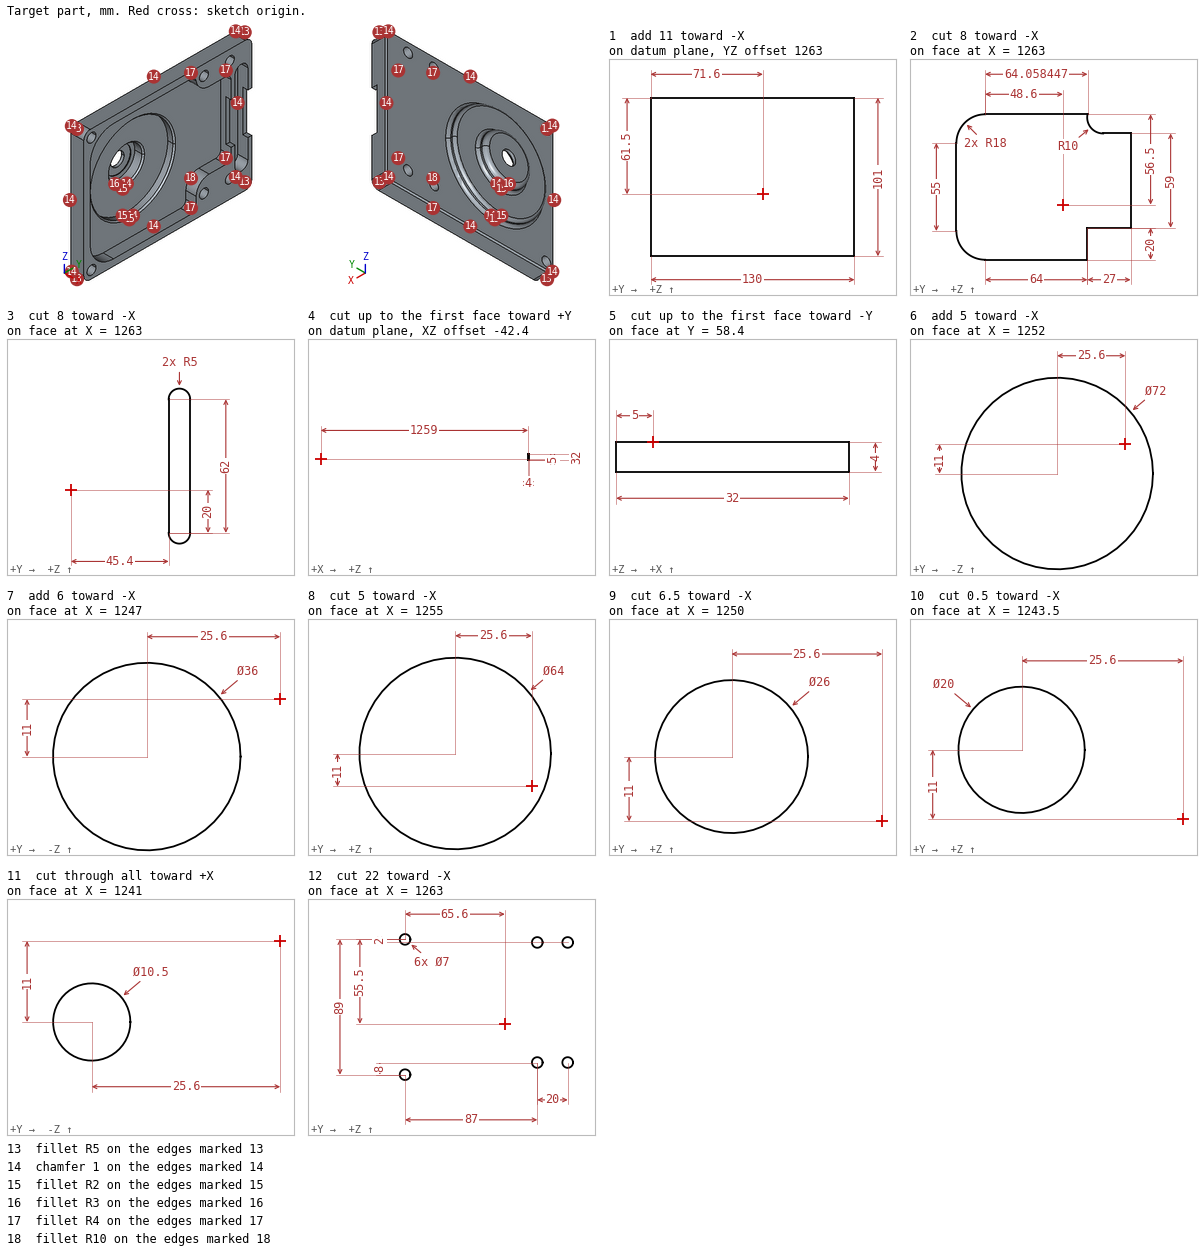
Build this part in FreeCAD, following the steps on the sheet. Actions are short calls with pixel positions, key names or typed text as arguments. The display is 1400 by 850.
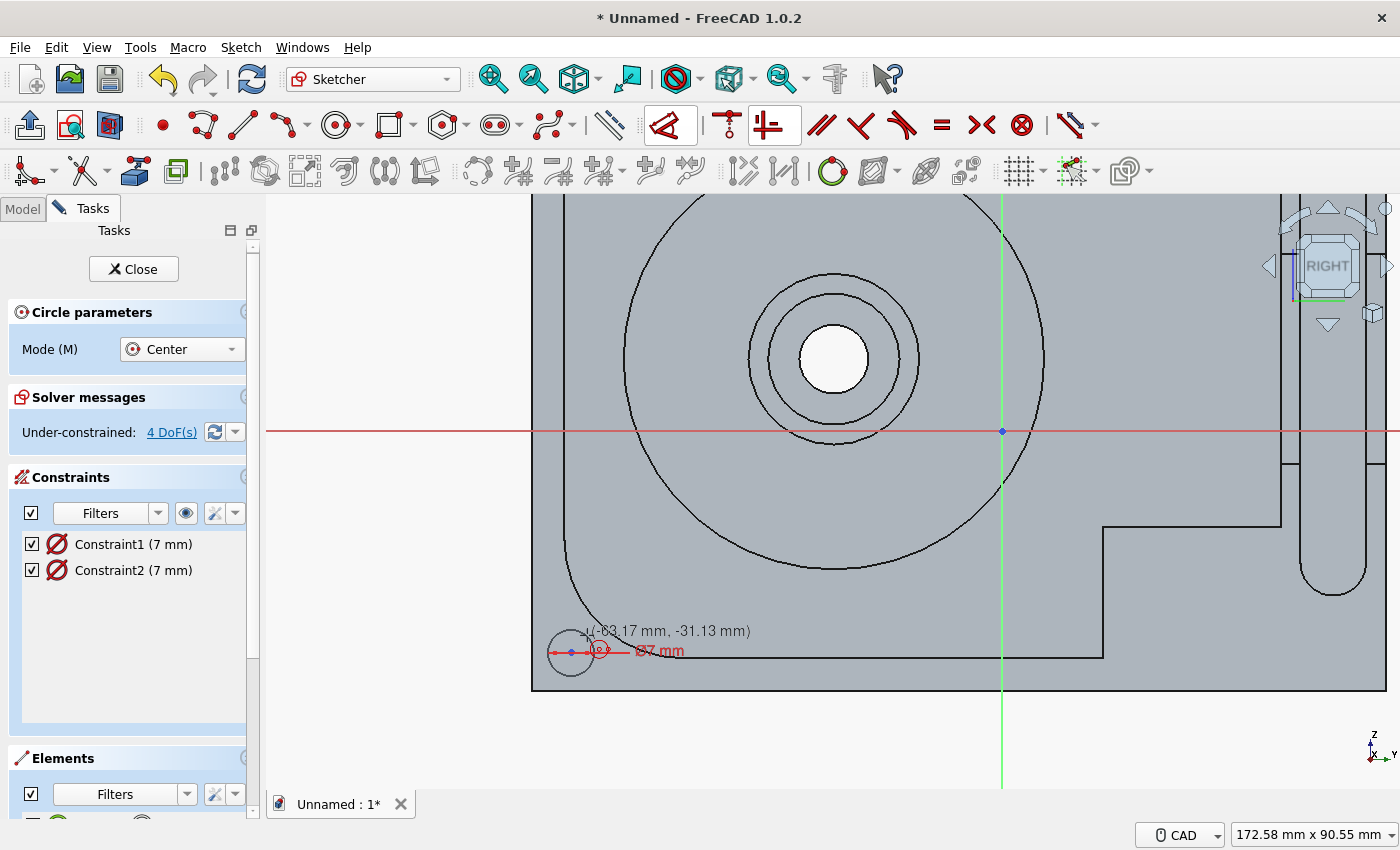
click(1143, 599)
move(1159, 583)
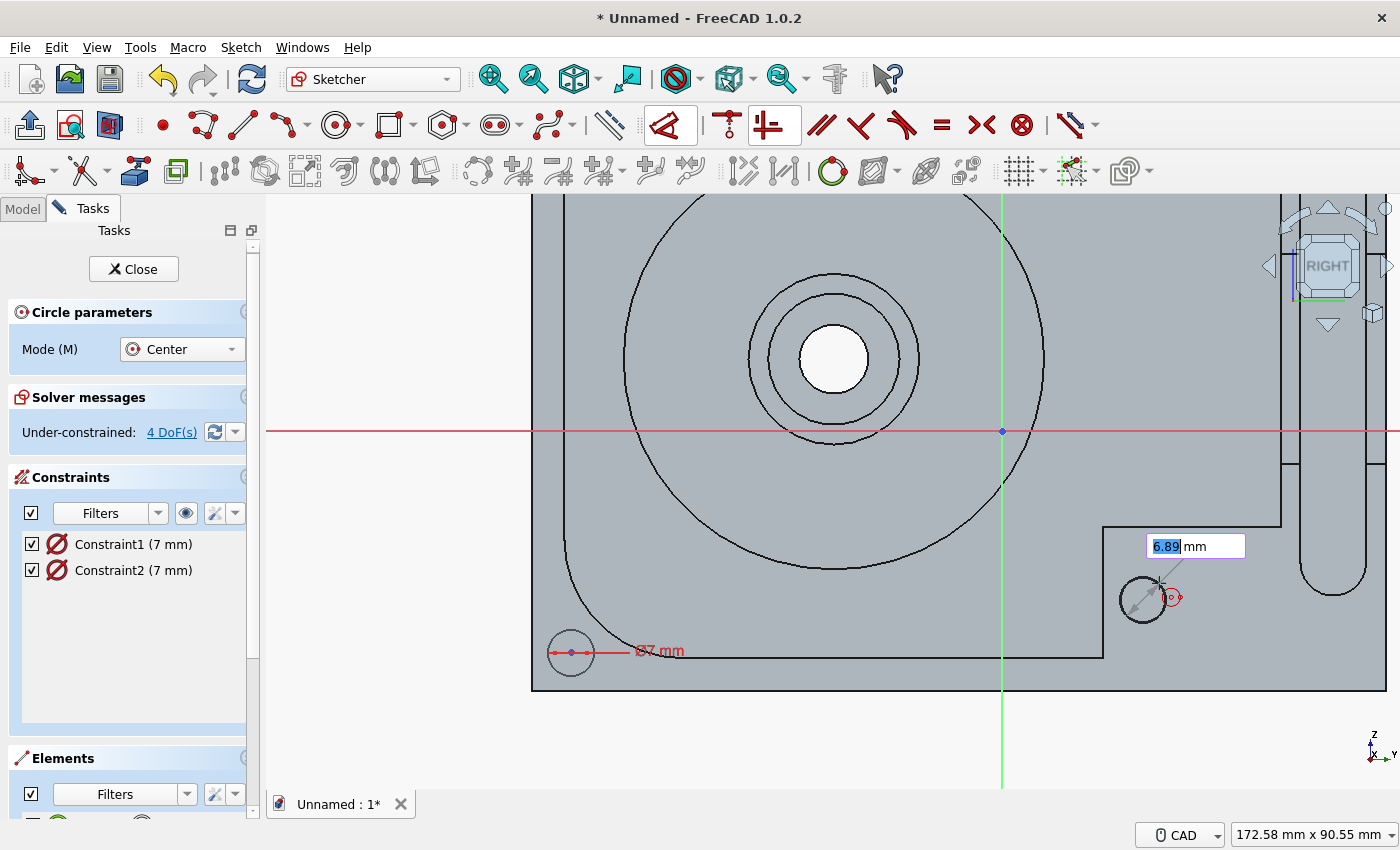
text(7)
key(Return)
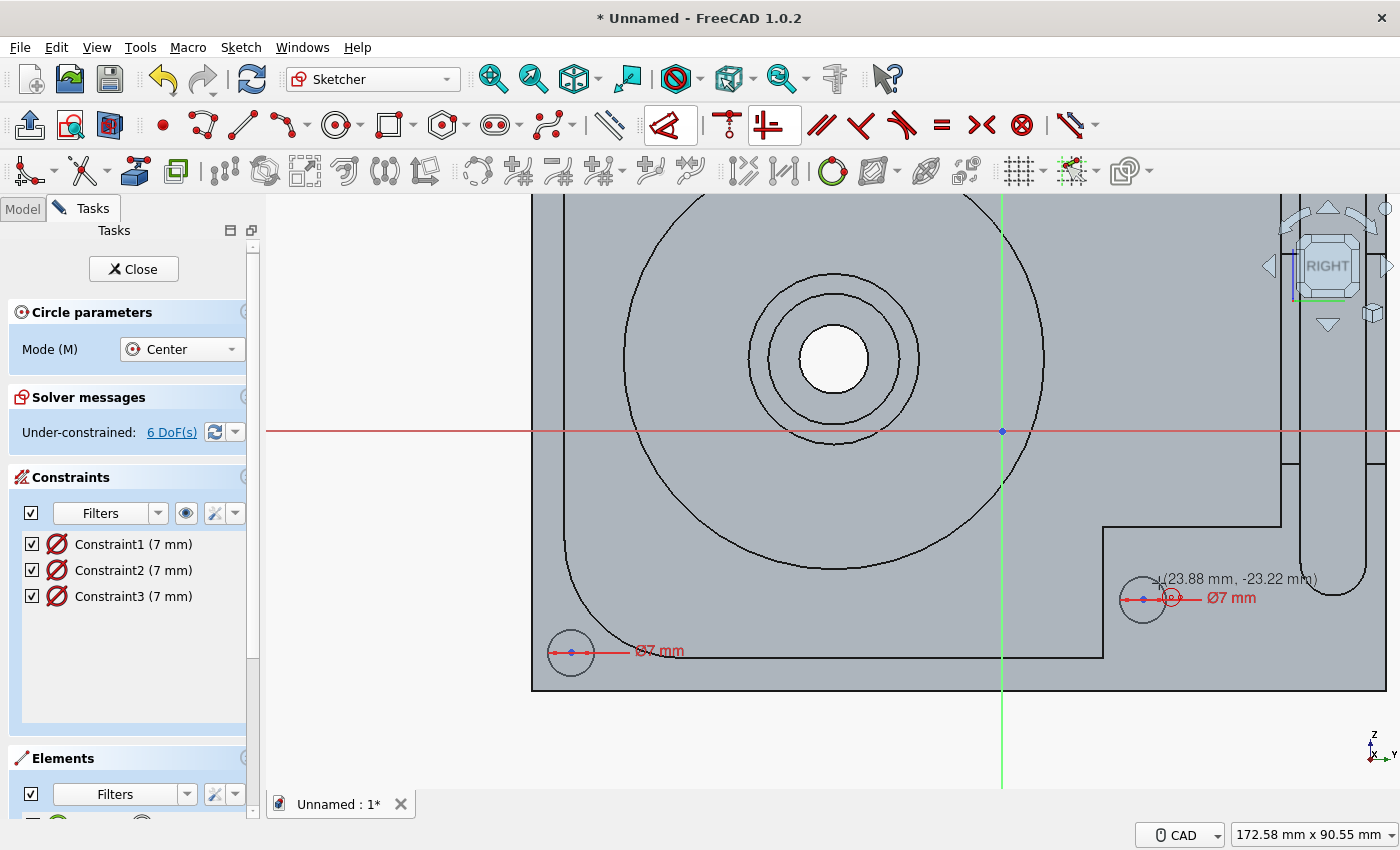
scroll(572, 652, down, 3)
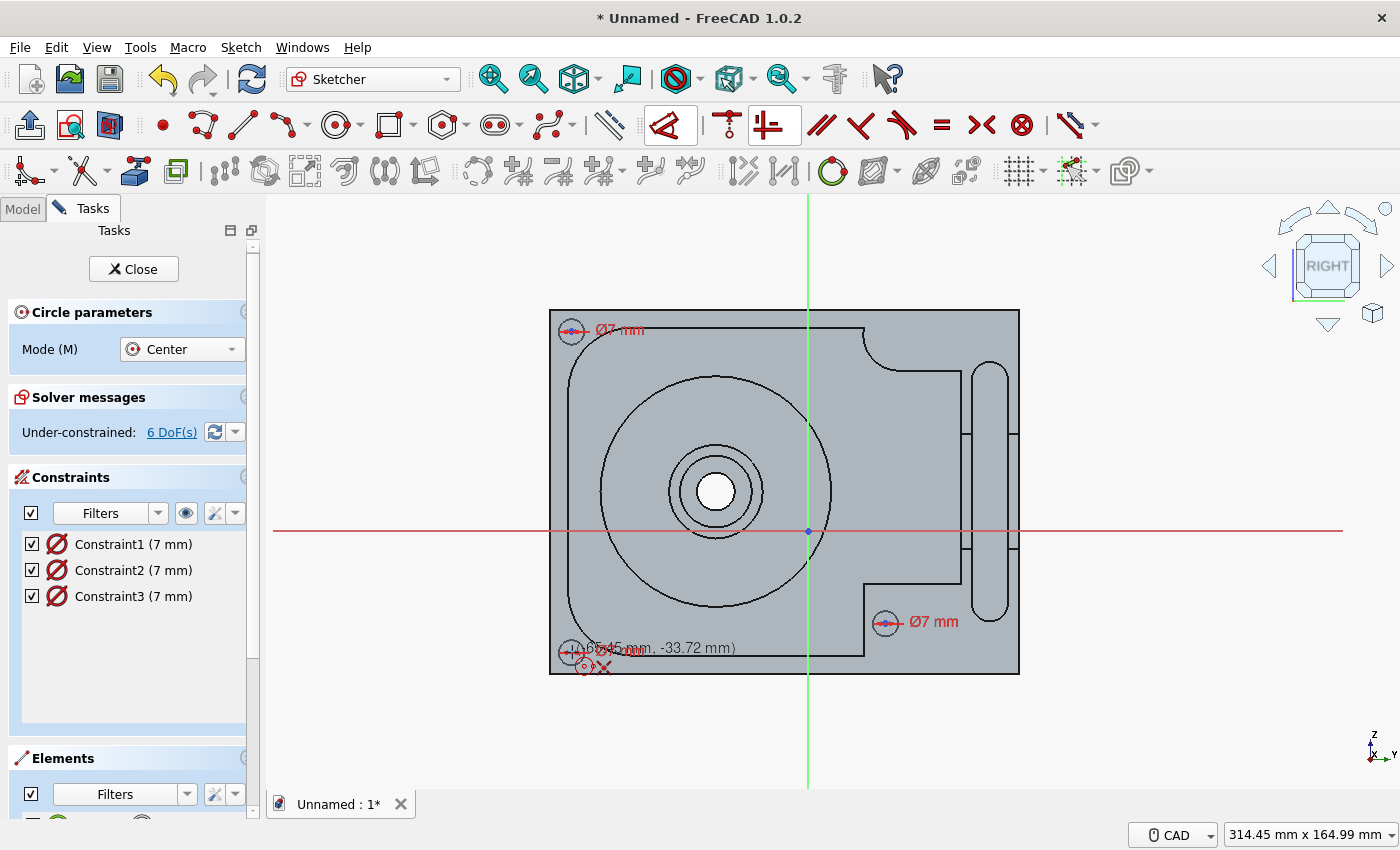
scroll(957, 623, up, 3)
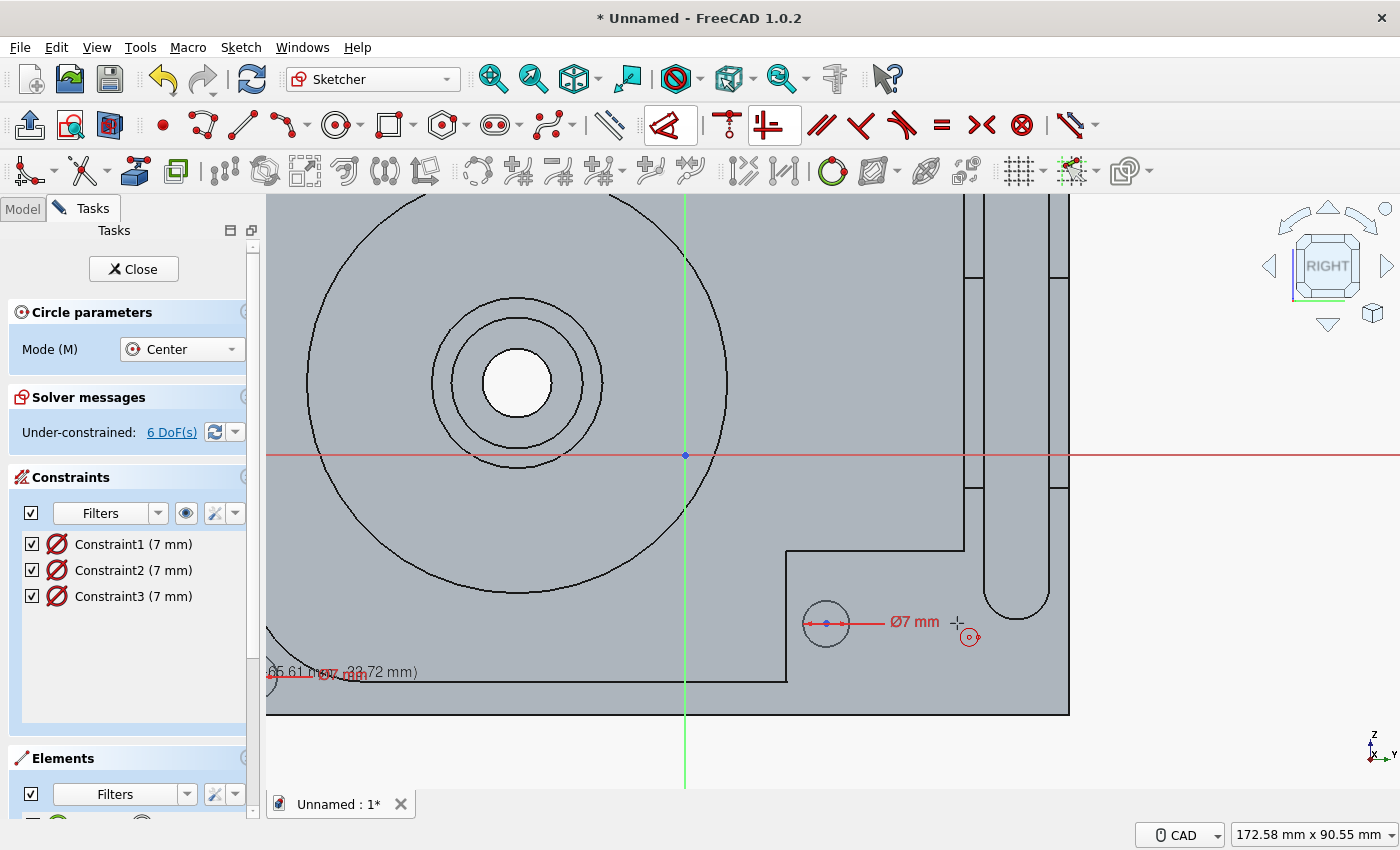
click(957, 623)
move(974, 607)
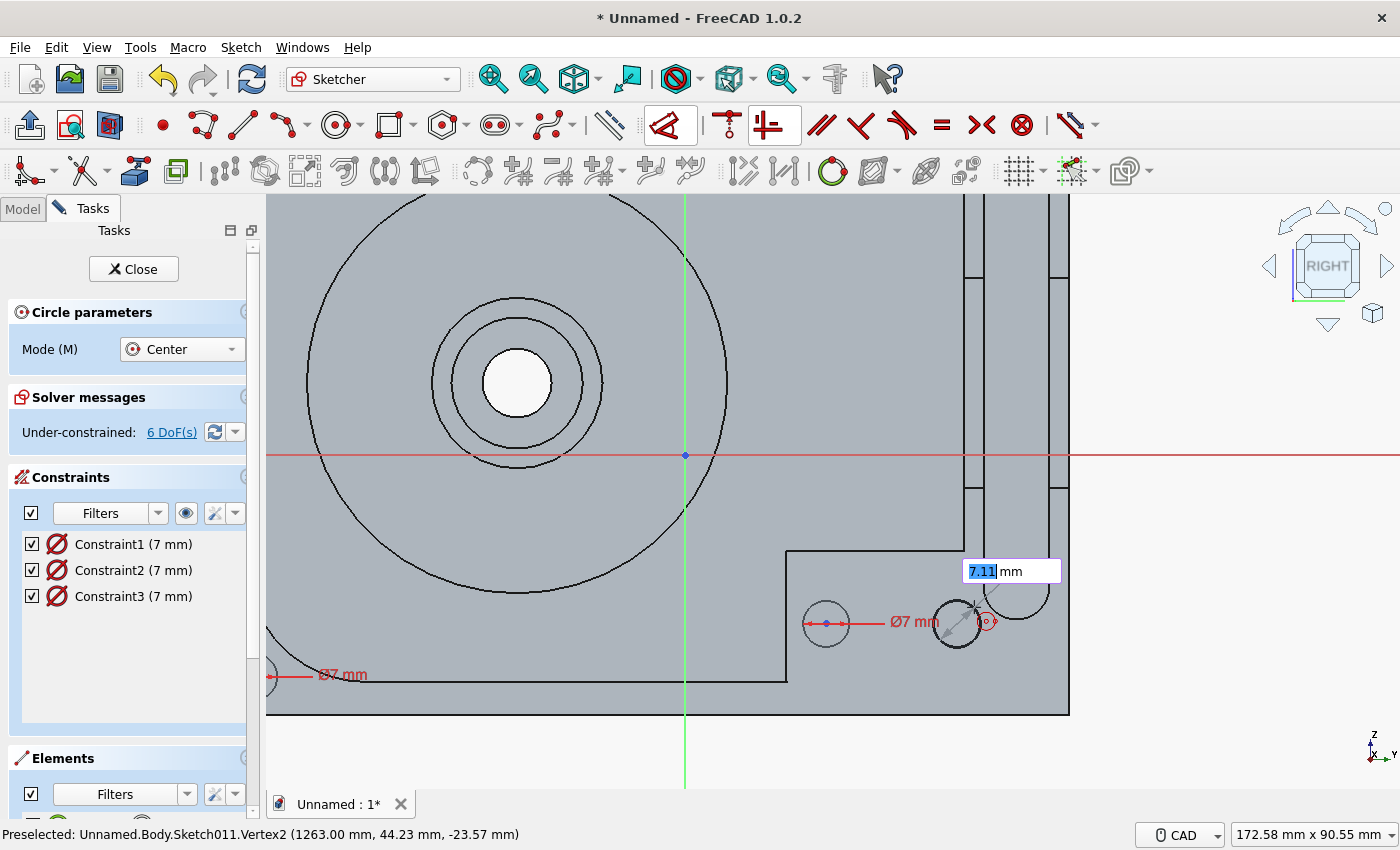
text(7)
key(Return)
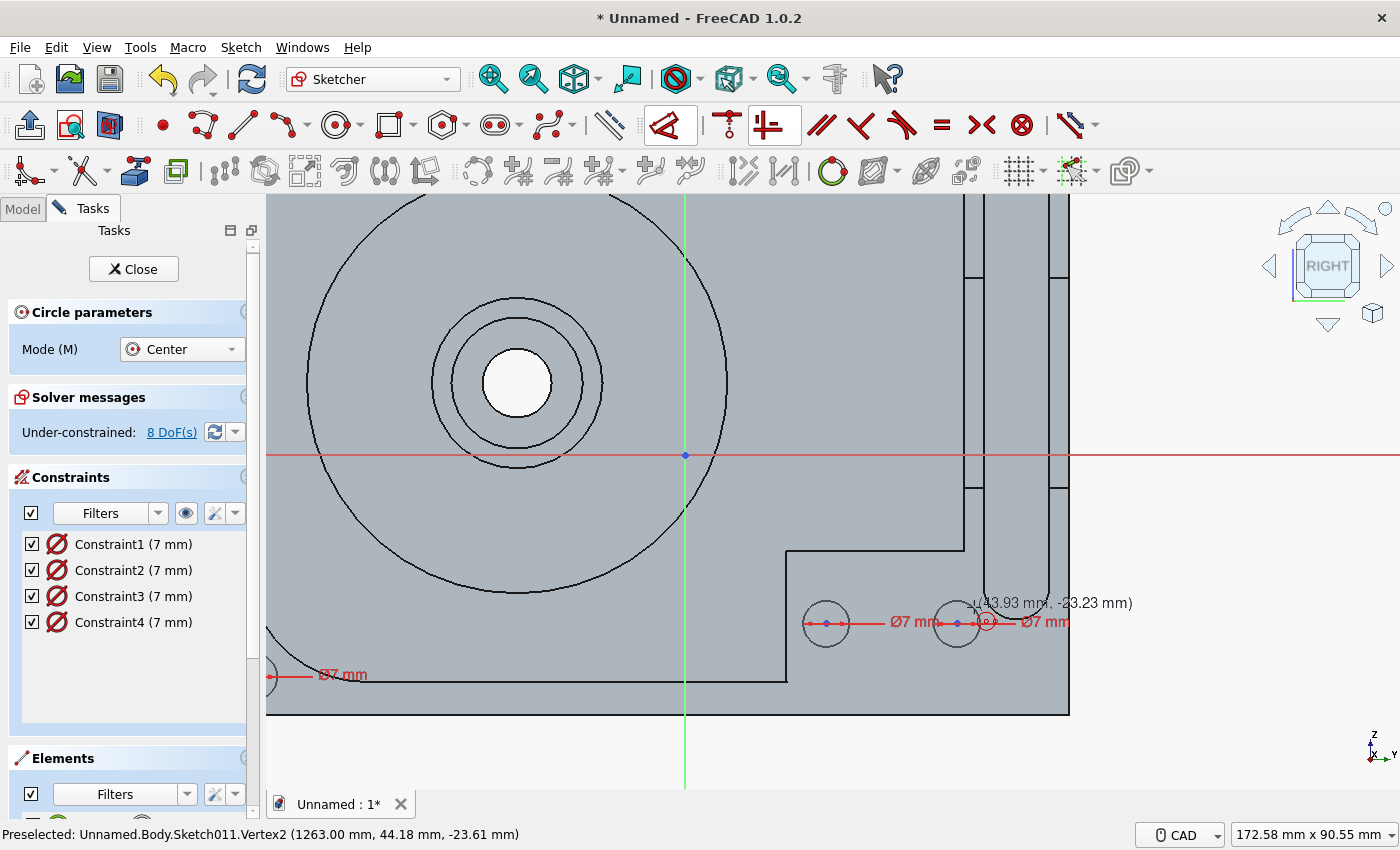
scroll(958, 623, down, 3)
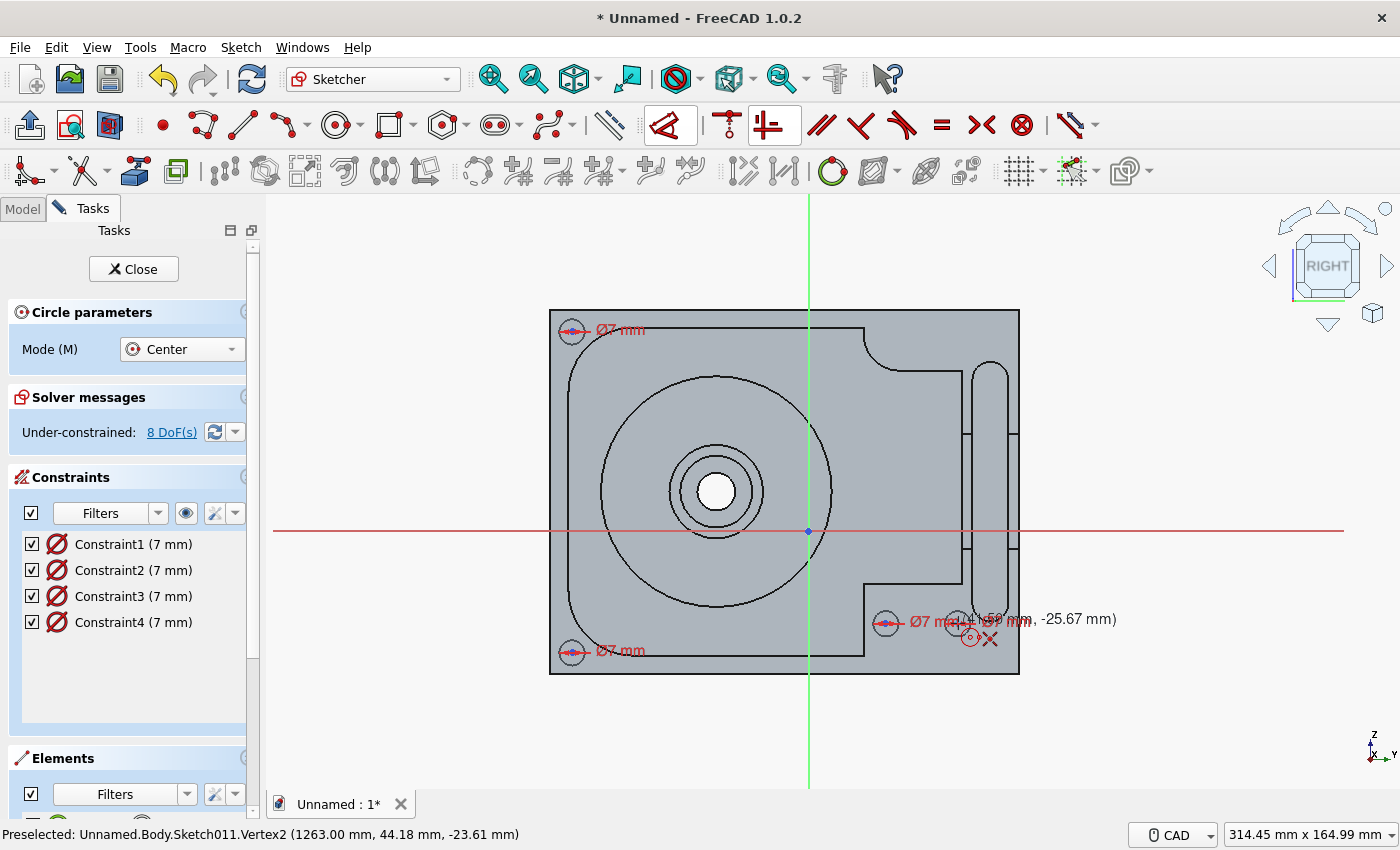
scroll(958, 338, up, 3)